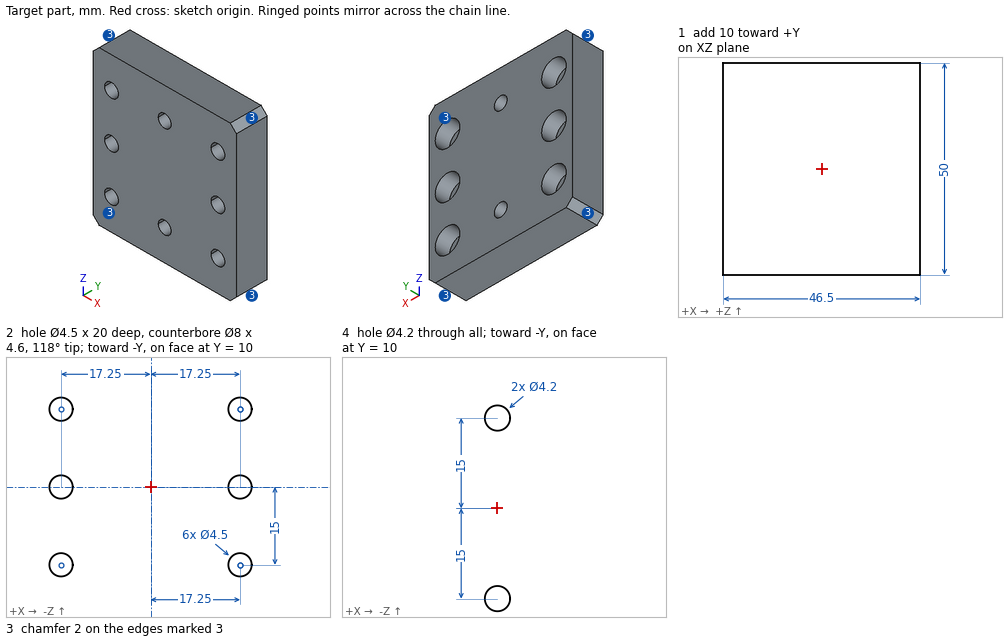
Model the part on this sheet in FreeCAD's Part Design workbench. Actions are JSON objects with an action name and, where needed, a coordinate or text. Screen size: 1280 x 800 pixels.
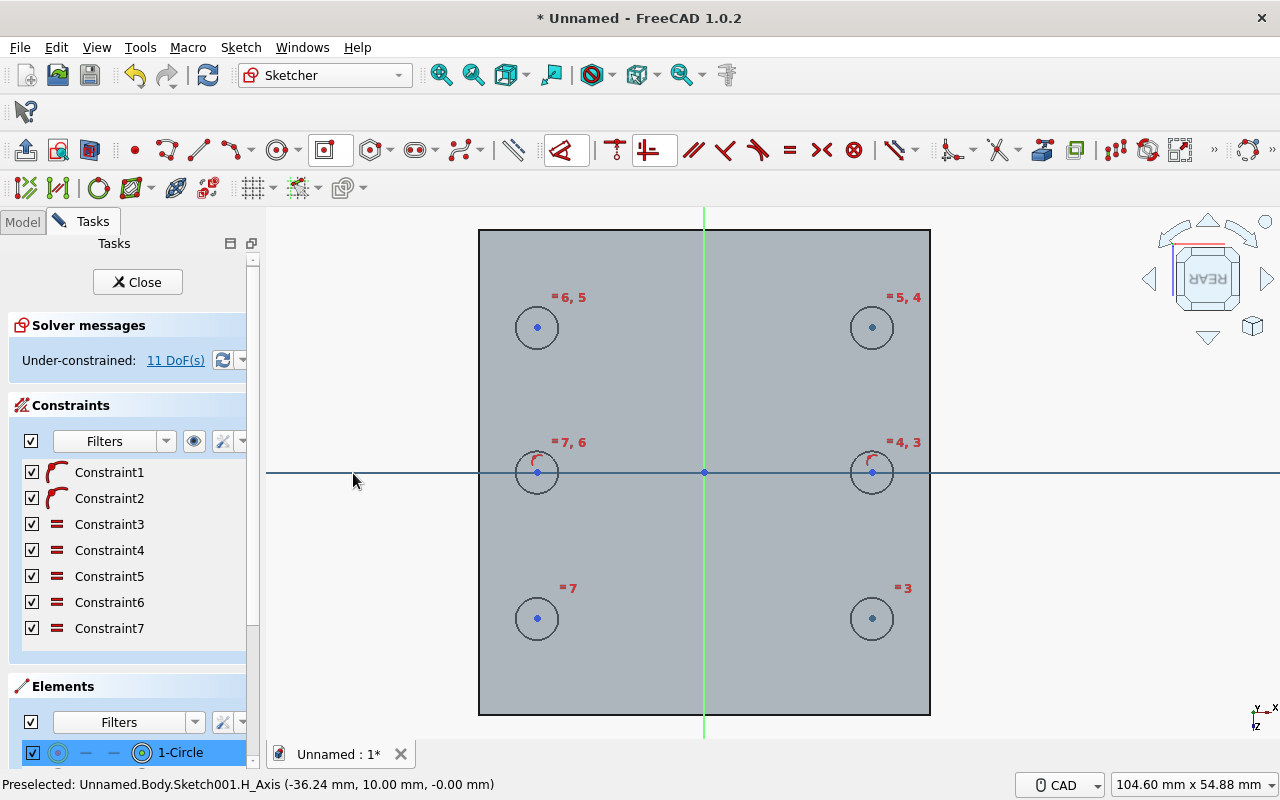
{"action": "left_click", "coordinate": [822, 150]}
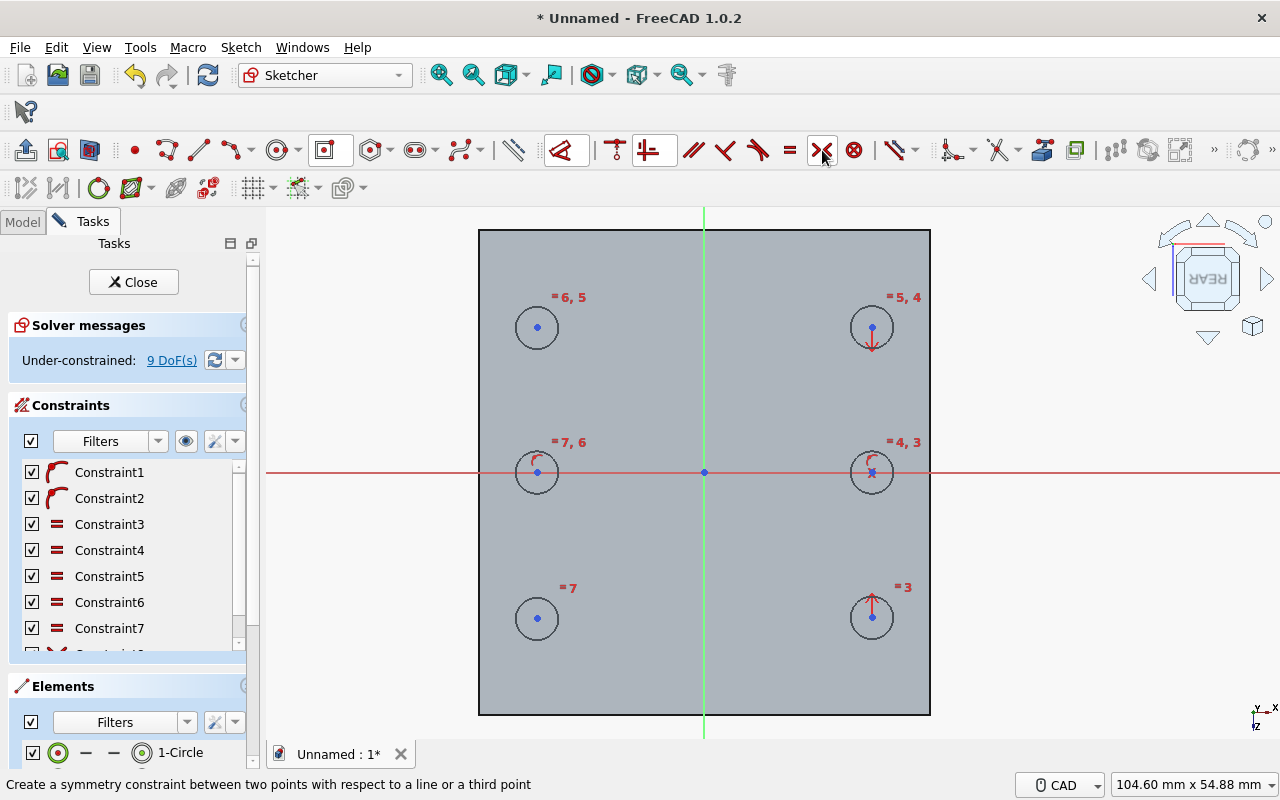
{"action": "left_click", "coordinate": [872, 327]}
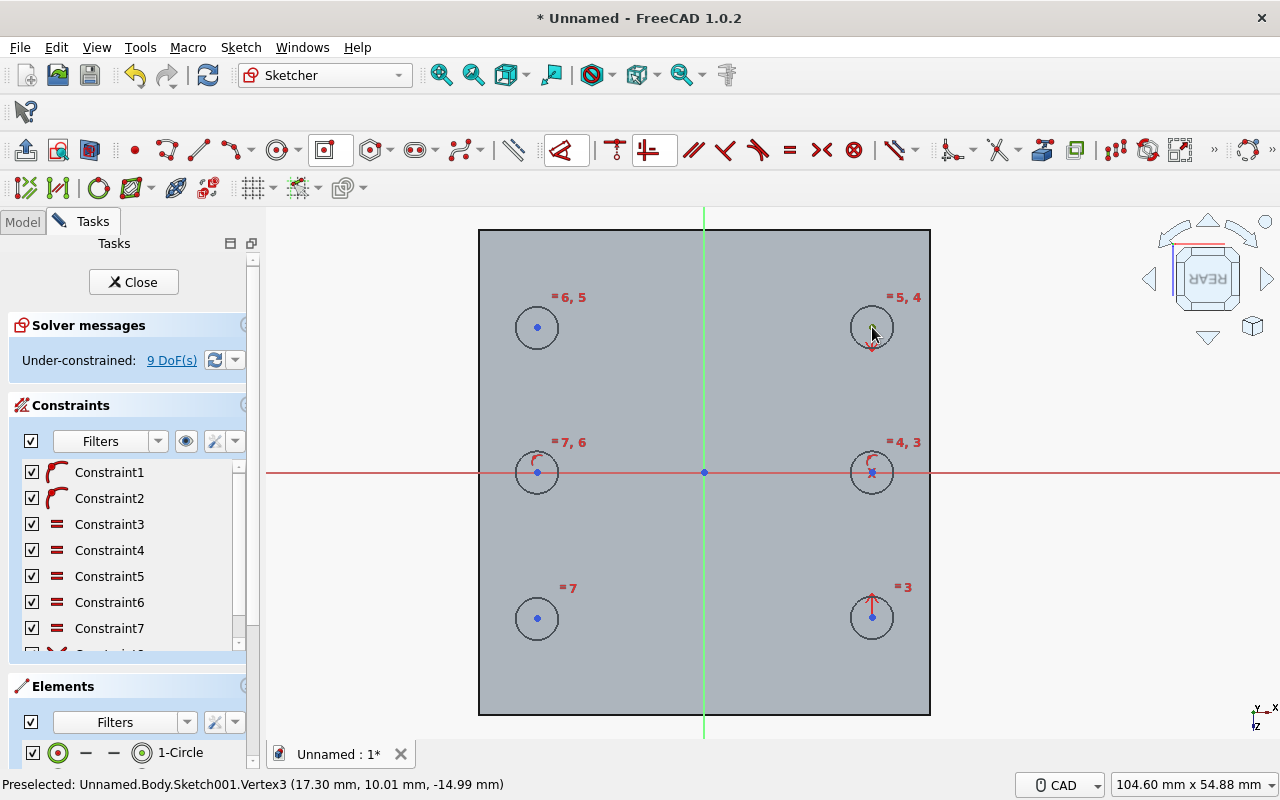
{"action": "left_click", "coordinate": [537, 328]}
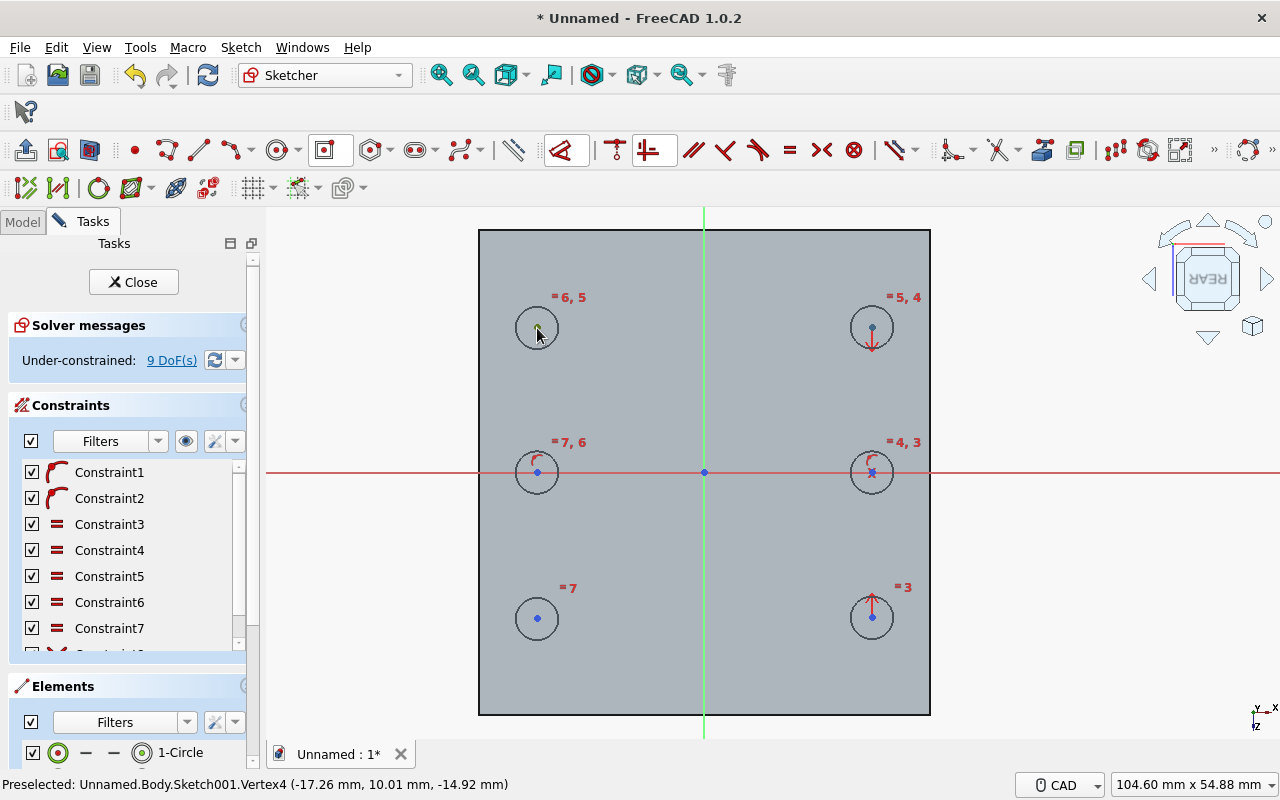
{"action": "left_click", "coordinate": [704, 677]}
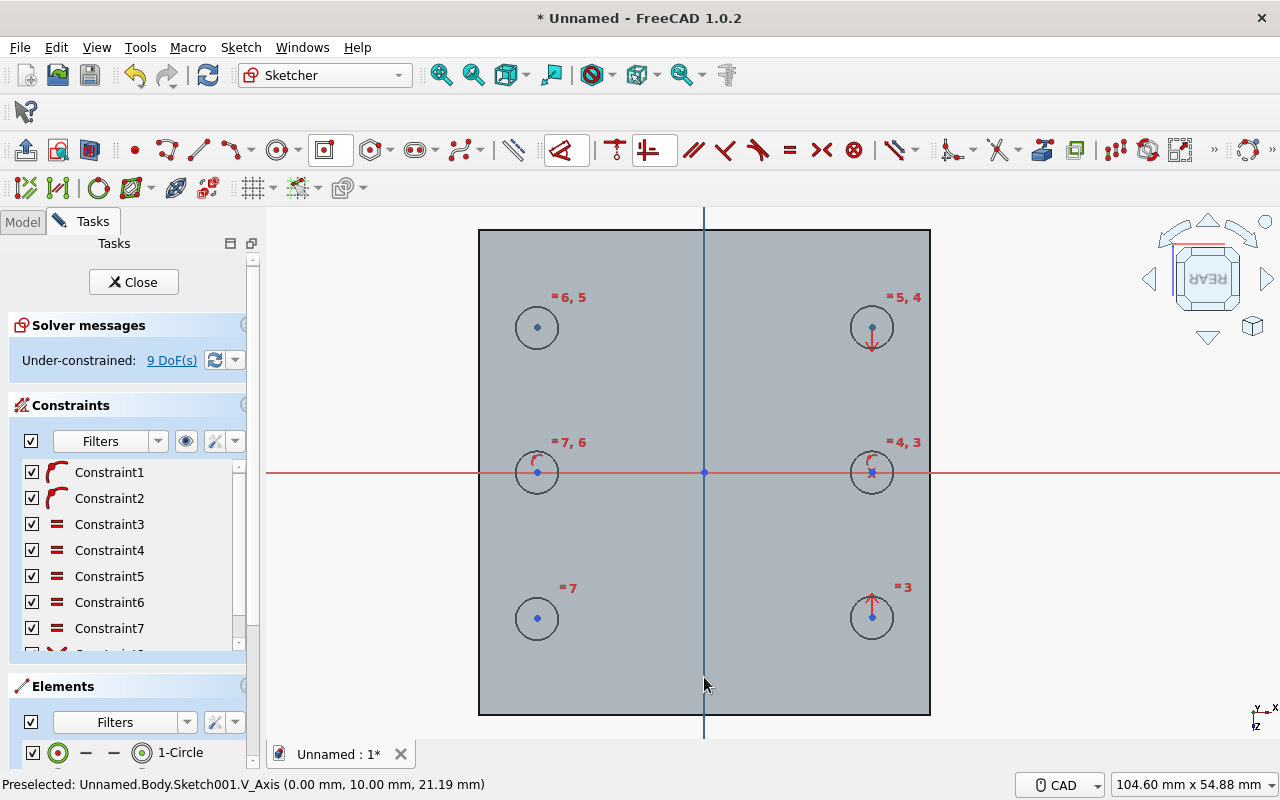
{"action": "key", "text": "s"}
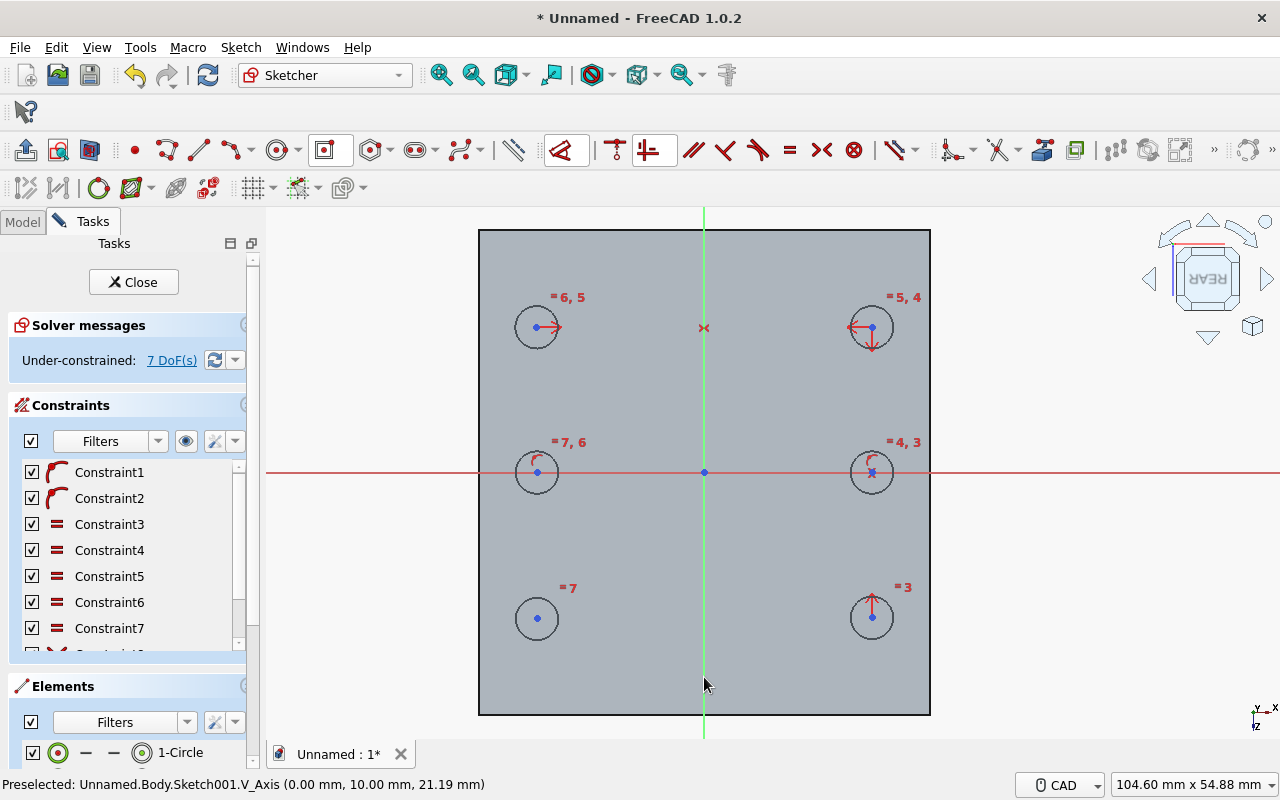
{"action": "left_click", "coordinate": [872, 618]}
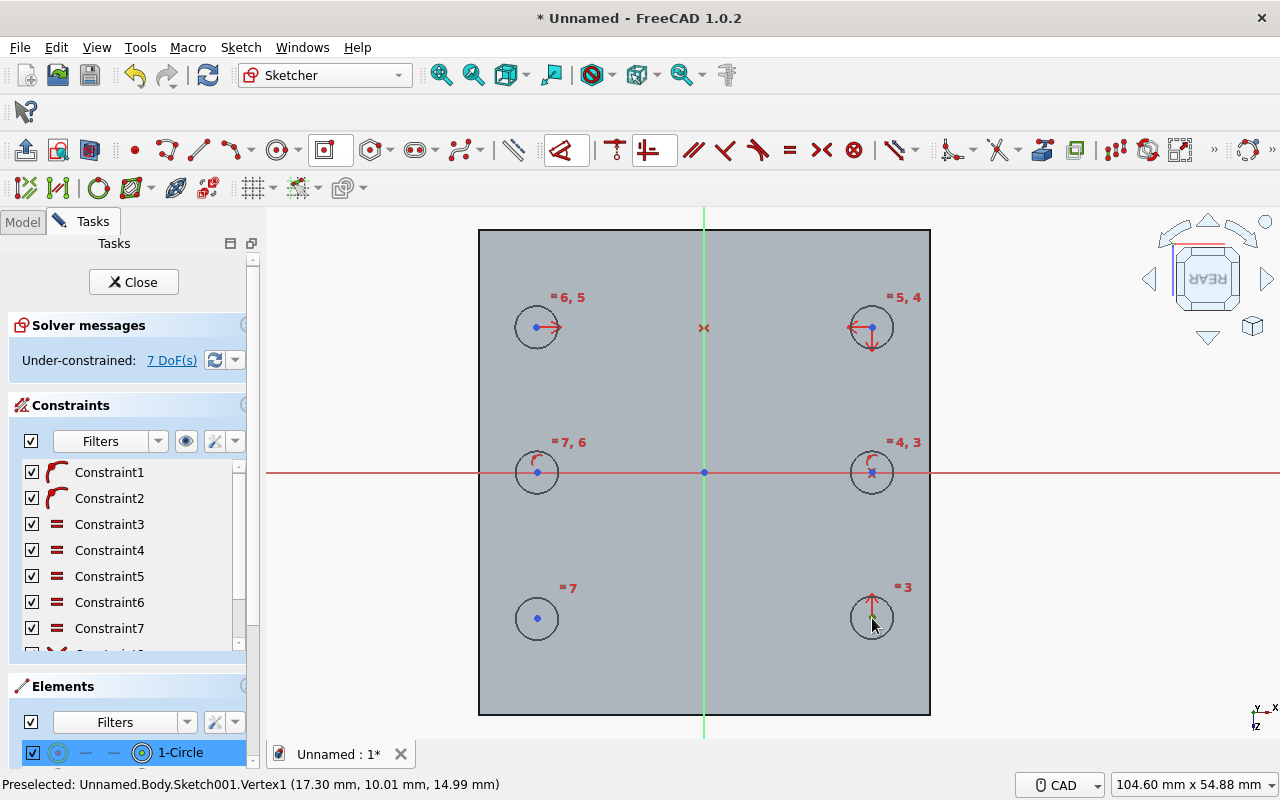
{"action": "left_click", "coordinate": [537, 619]}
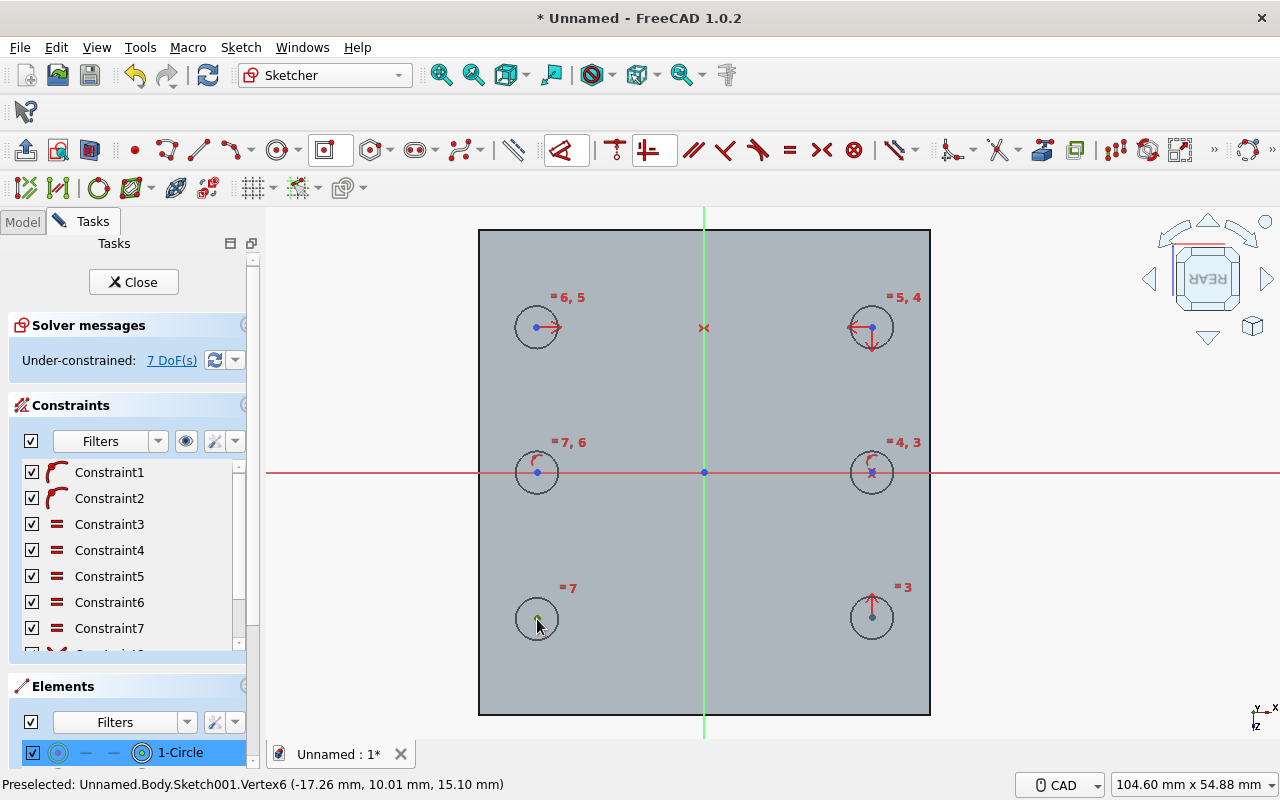
{"action": "left_click", "coordinate": [704, 677]}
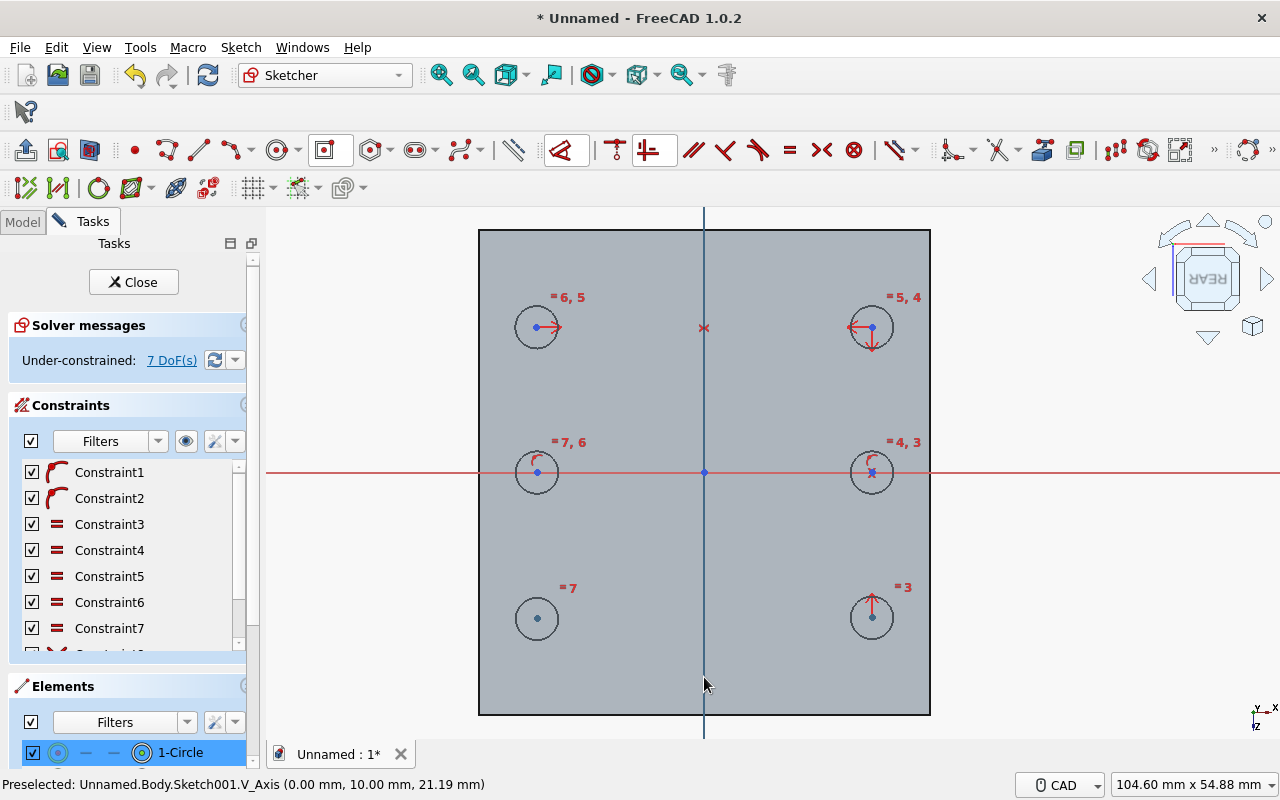
{"action": "key", "text": "s"}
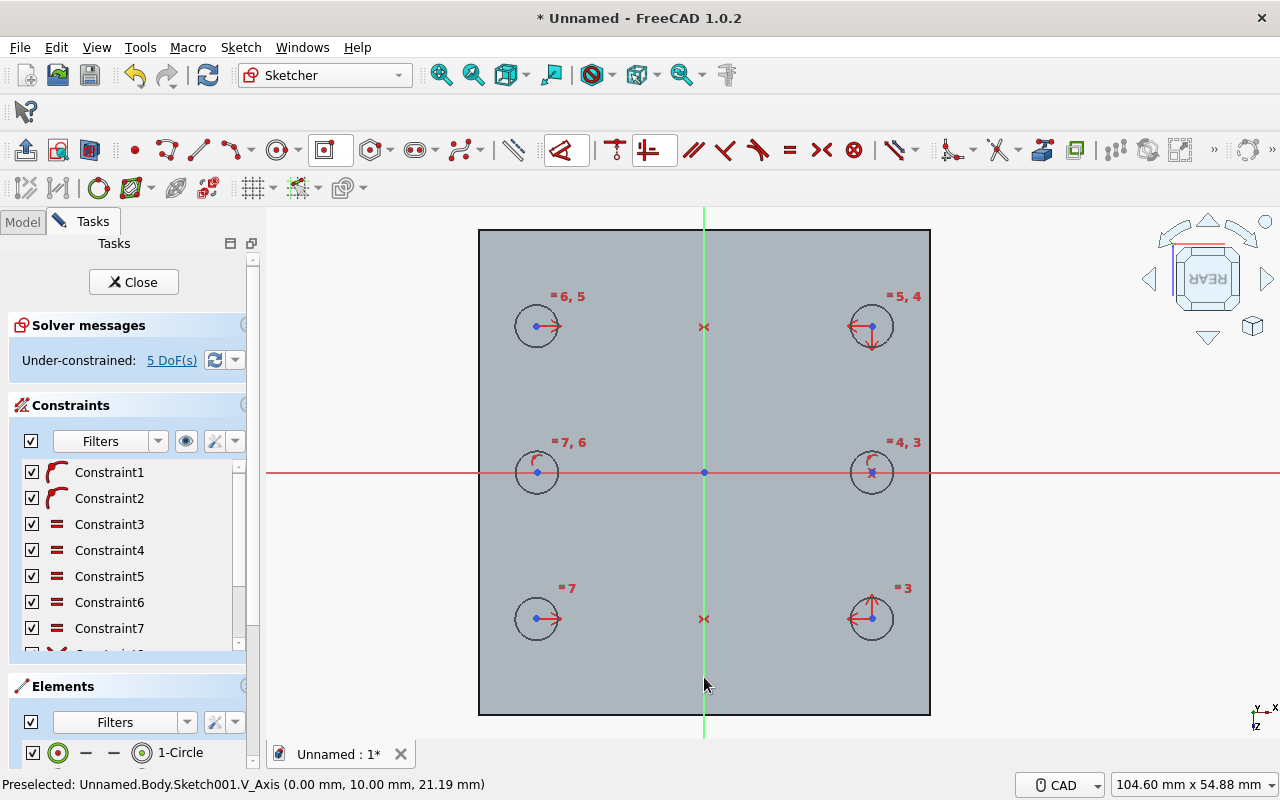
{"action": "left_click", "coordinate": [887, 604]}